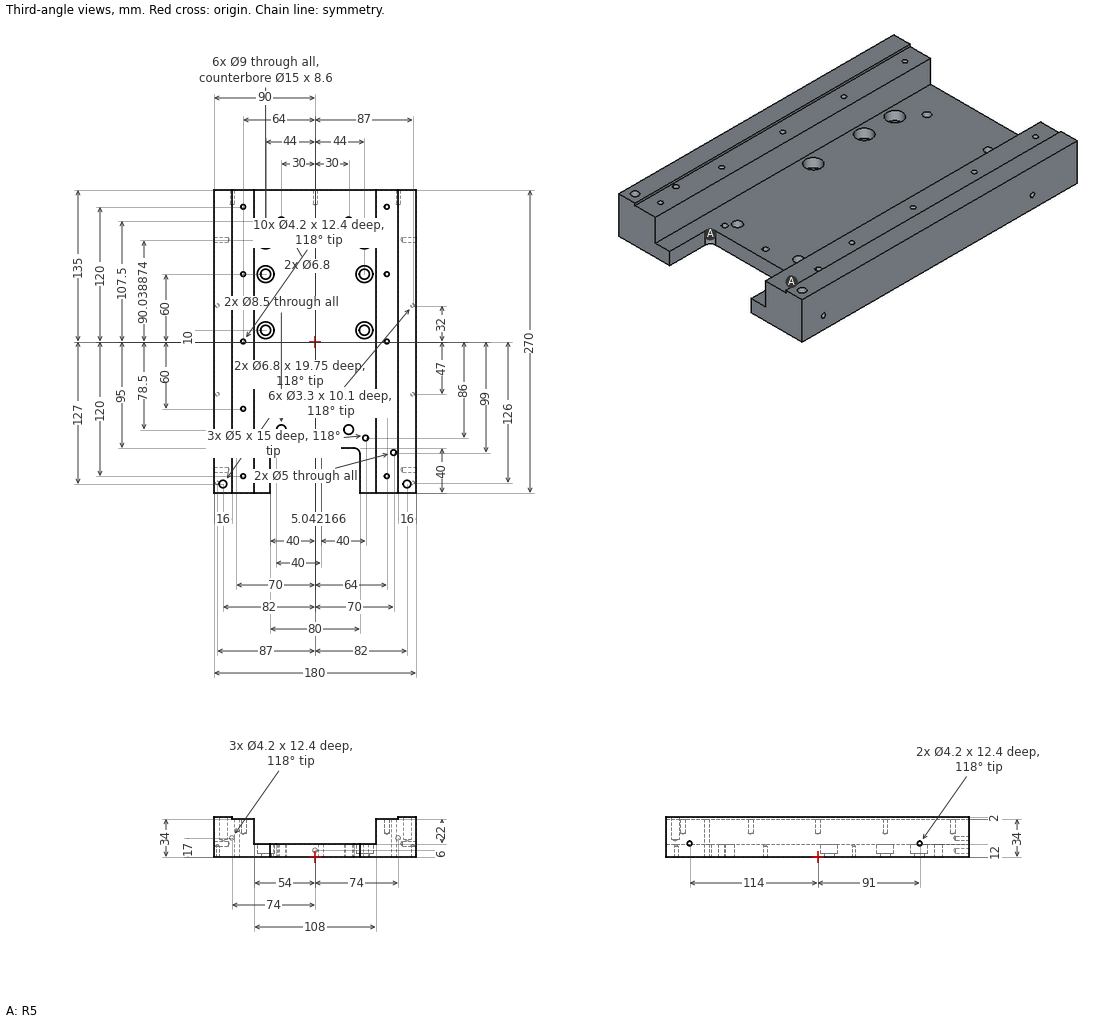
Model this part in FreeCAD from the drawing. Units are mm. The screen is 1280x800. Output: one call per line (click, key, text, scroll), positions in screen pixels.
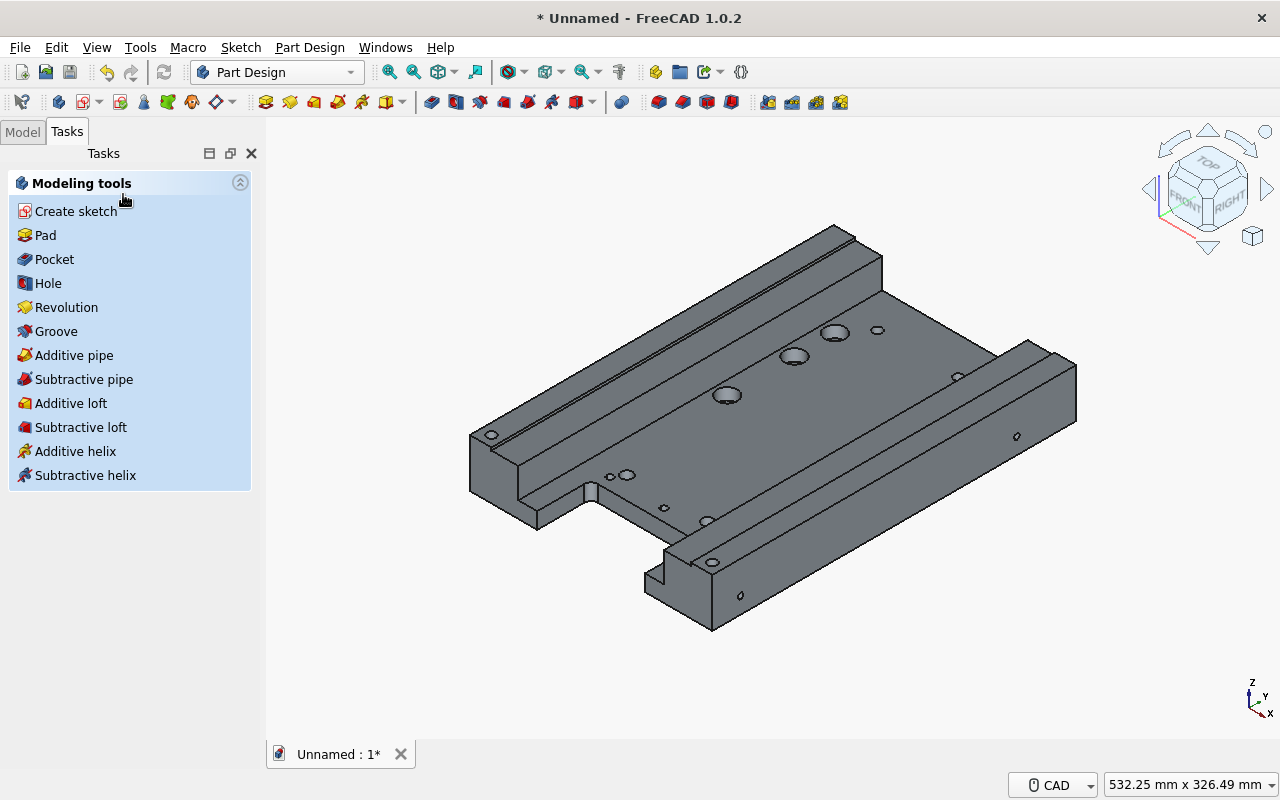
click(456, 102)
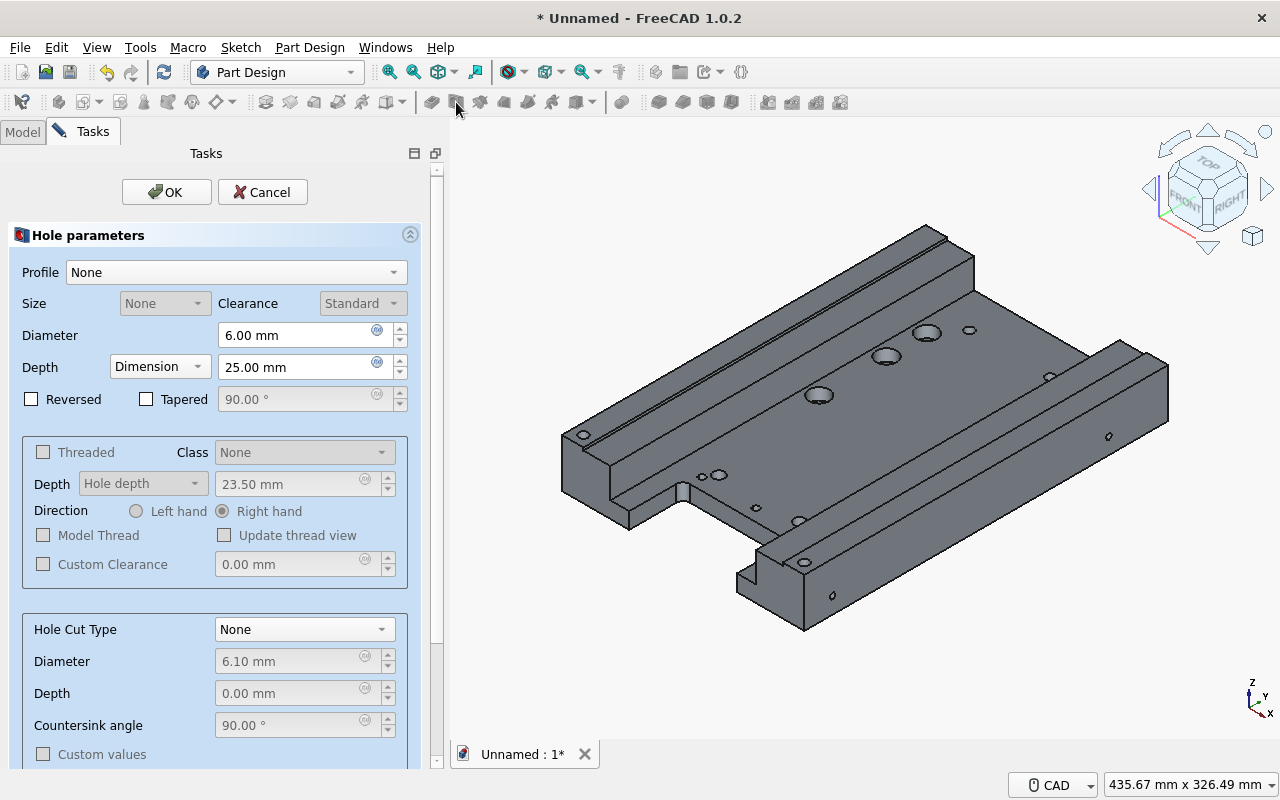
triple_click(305, 335)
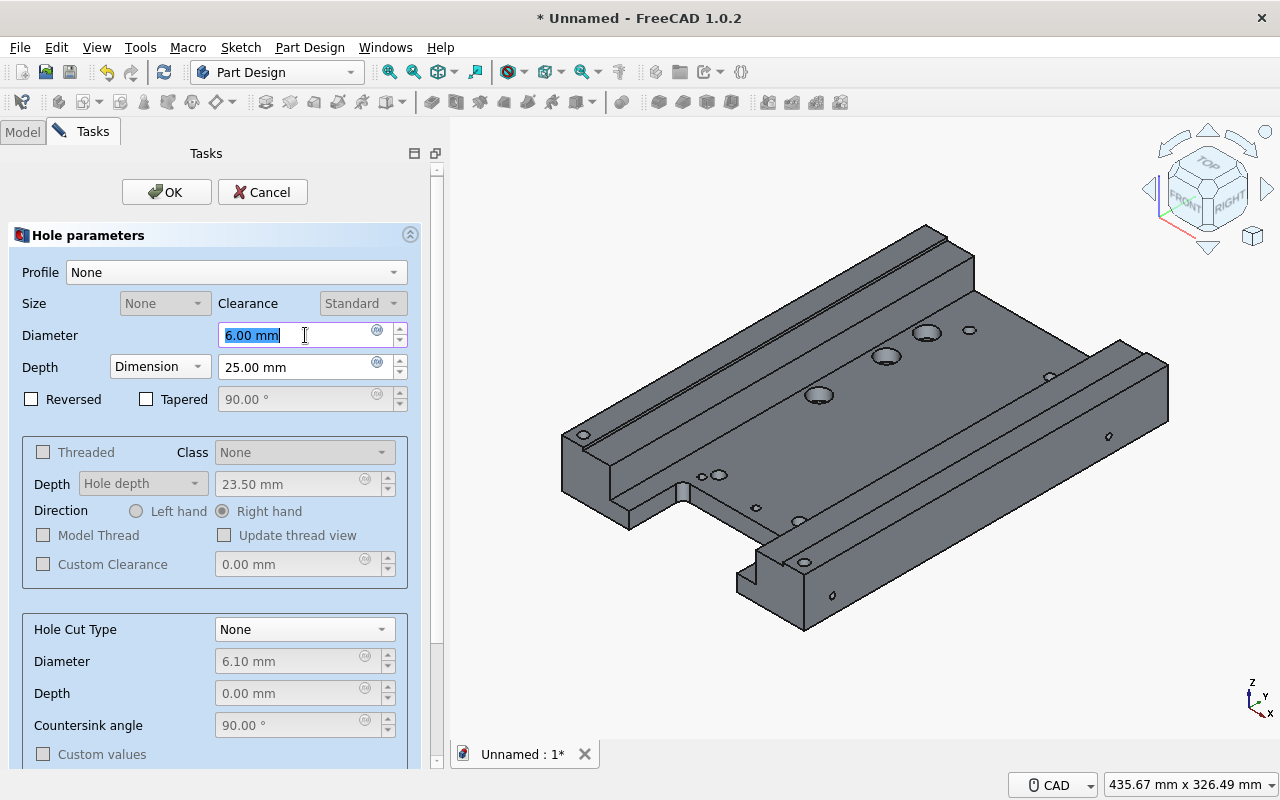
text(5)
key(Tab)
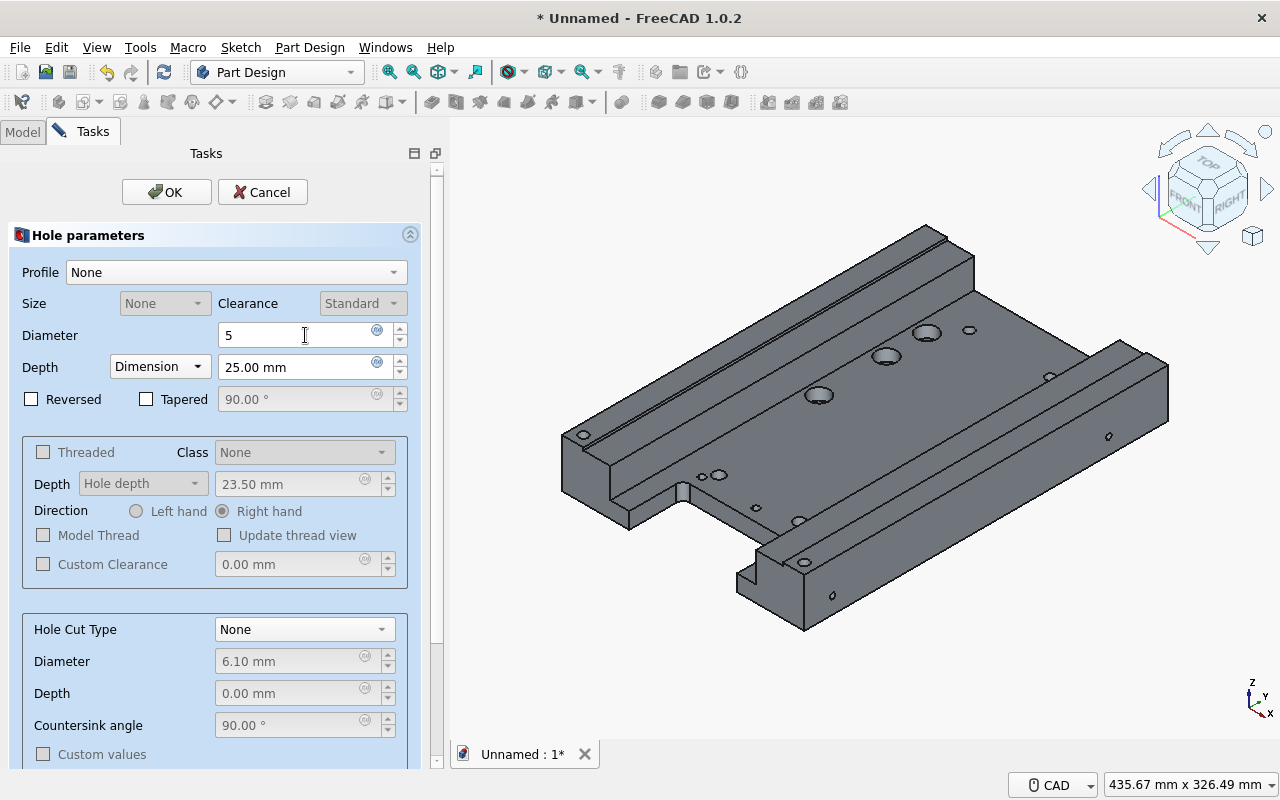
click(161, 366)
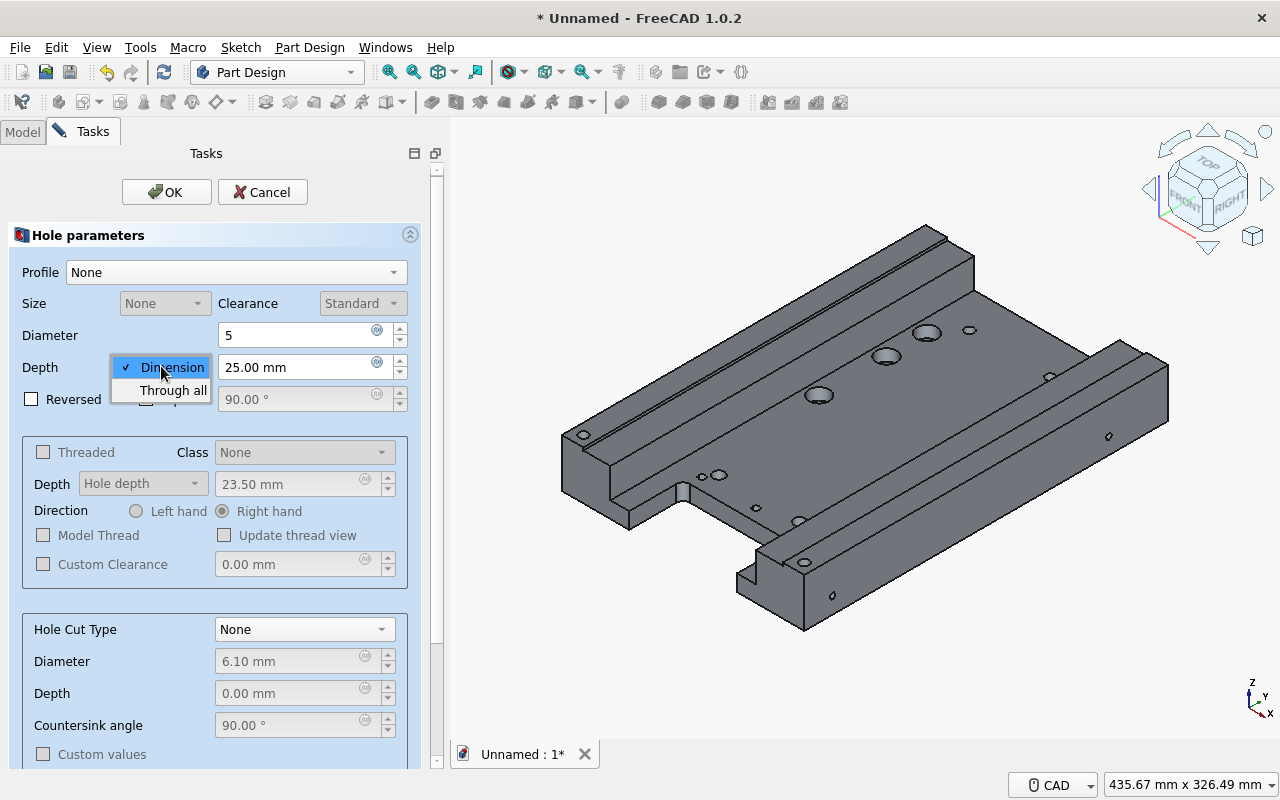
click(160, 390)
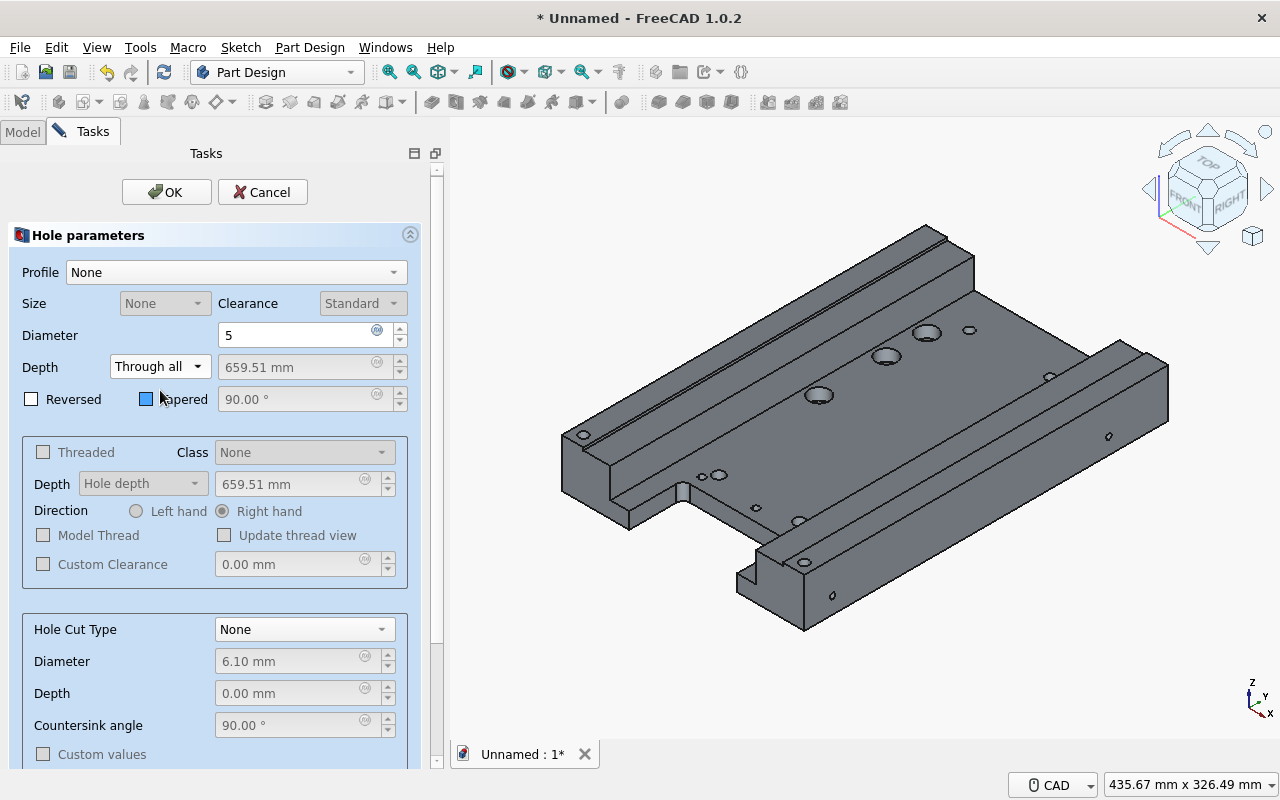
click(30, 399)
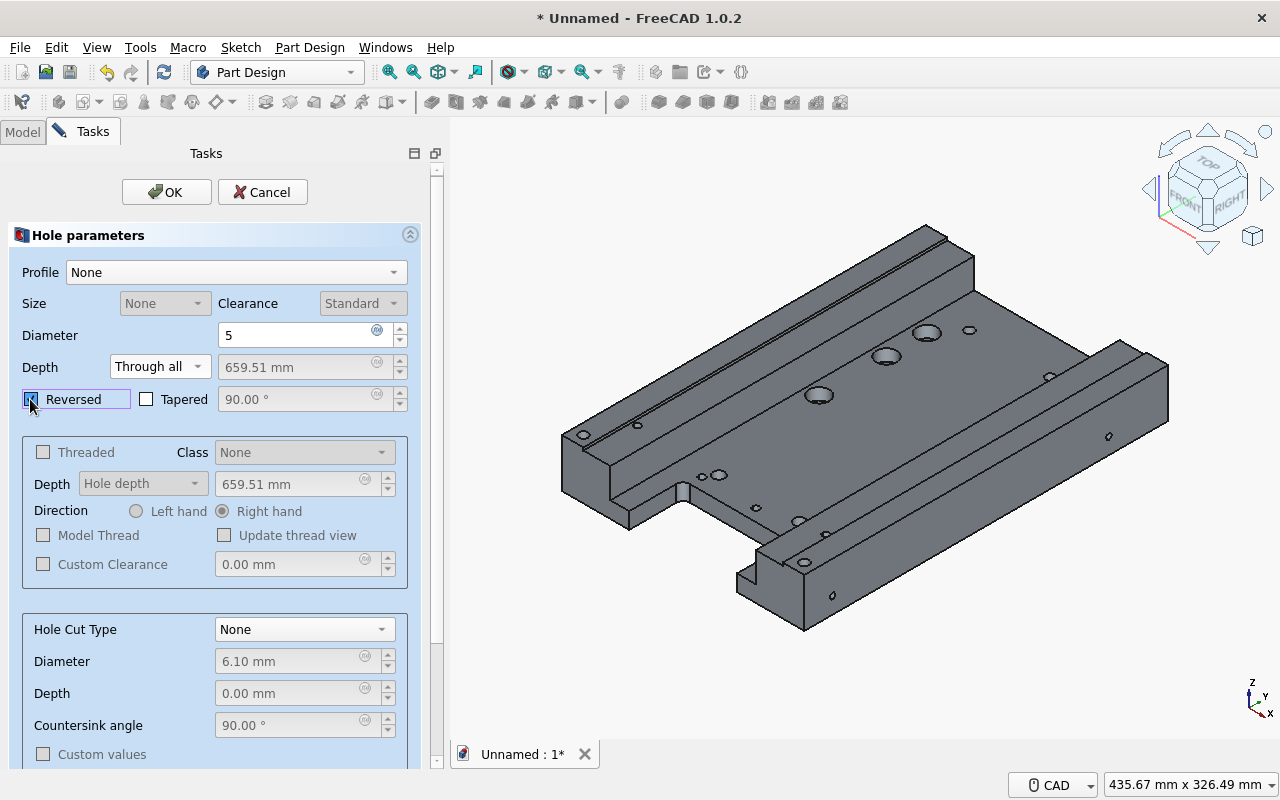
click(167, 192)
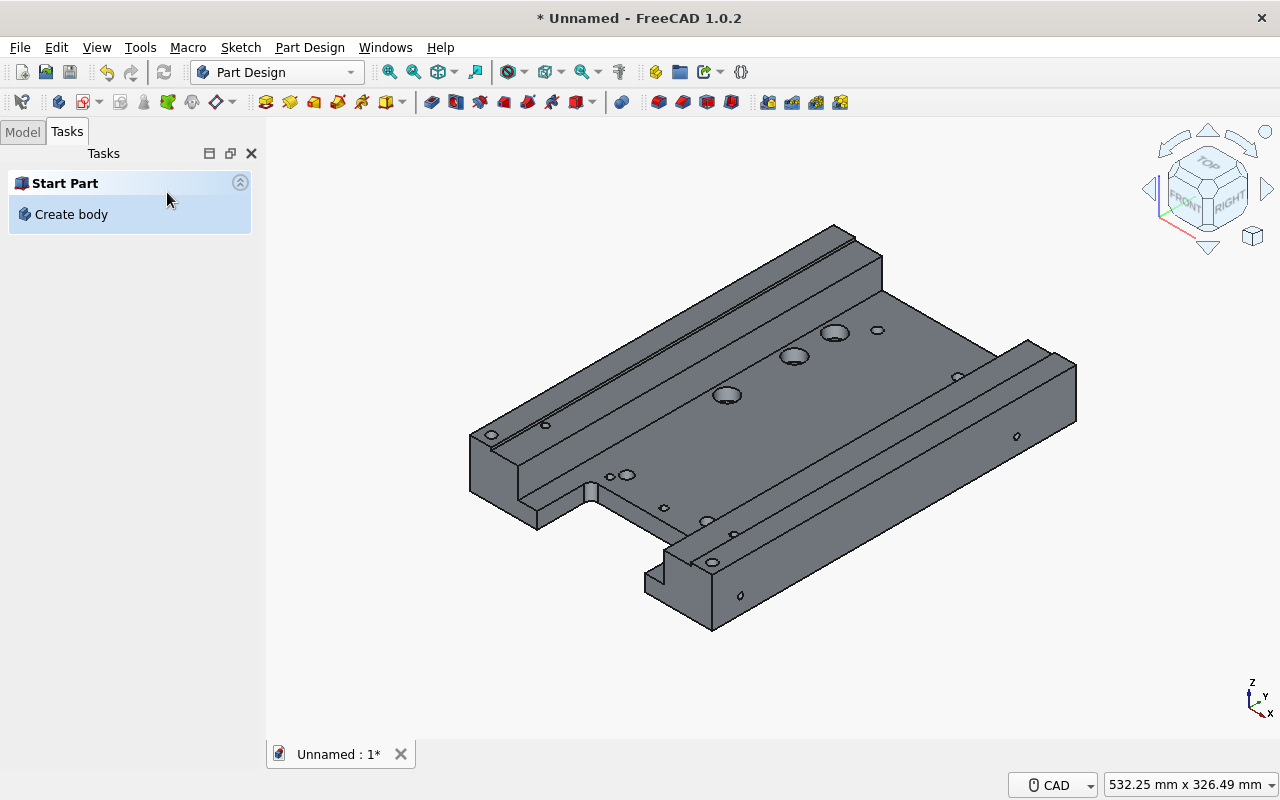
click(84, 102)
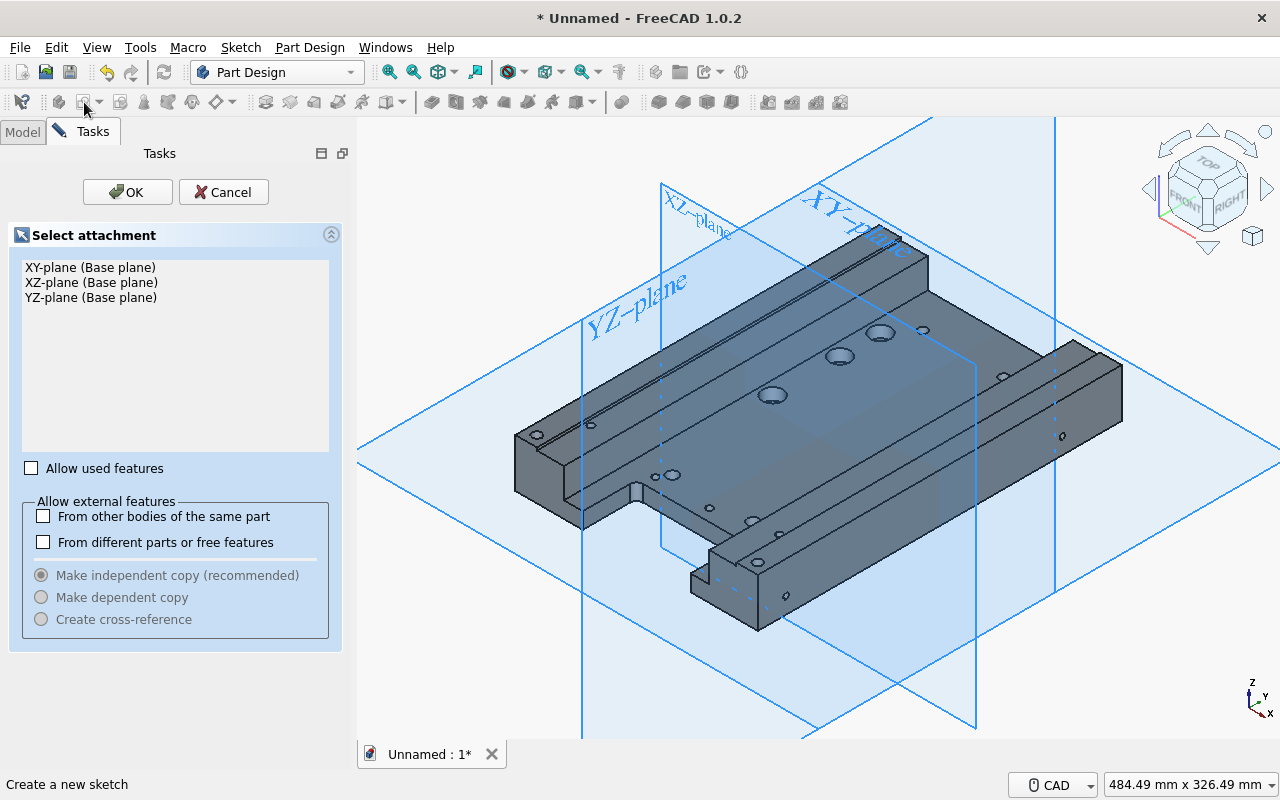
click(82, 268)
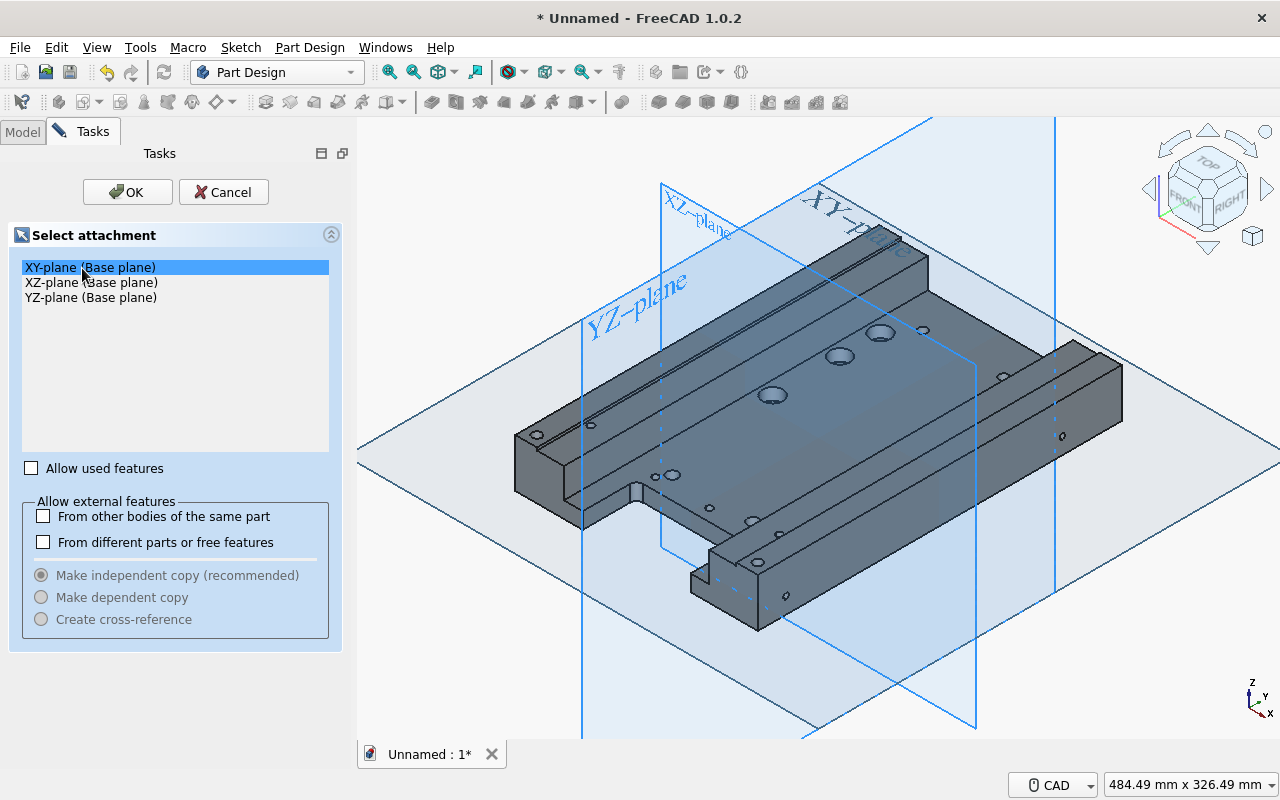
click(128, 192)